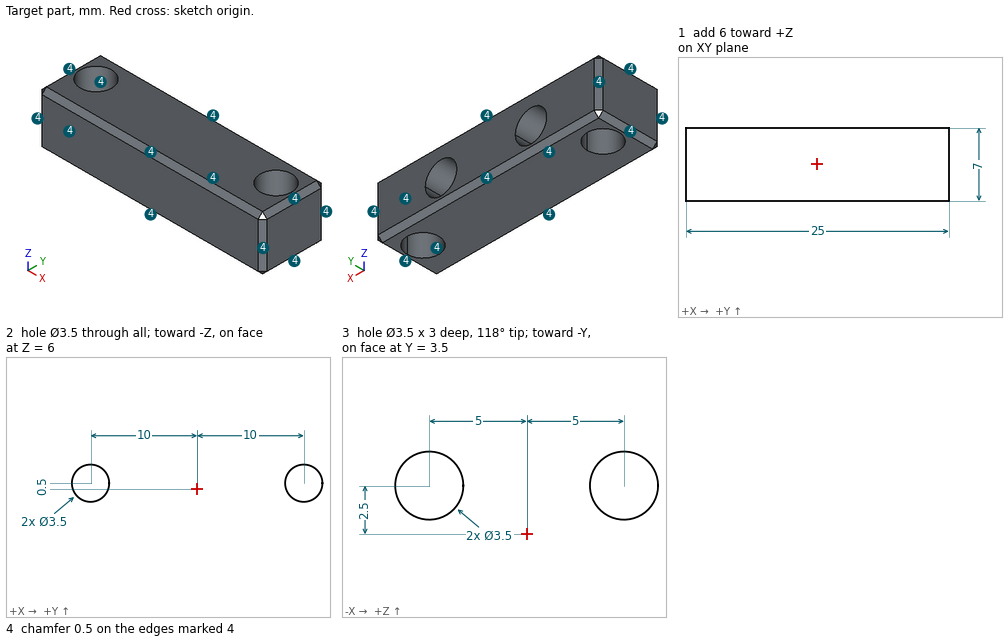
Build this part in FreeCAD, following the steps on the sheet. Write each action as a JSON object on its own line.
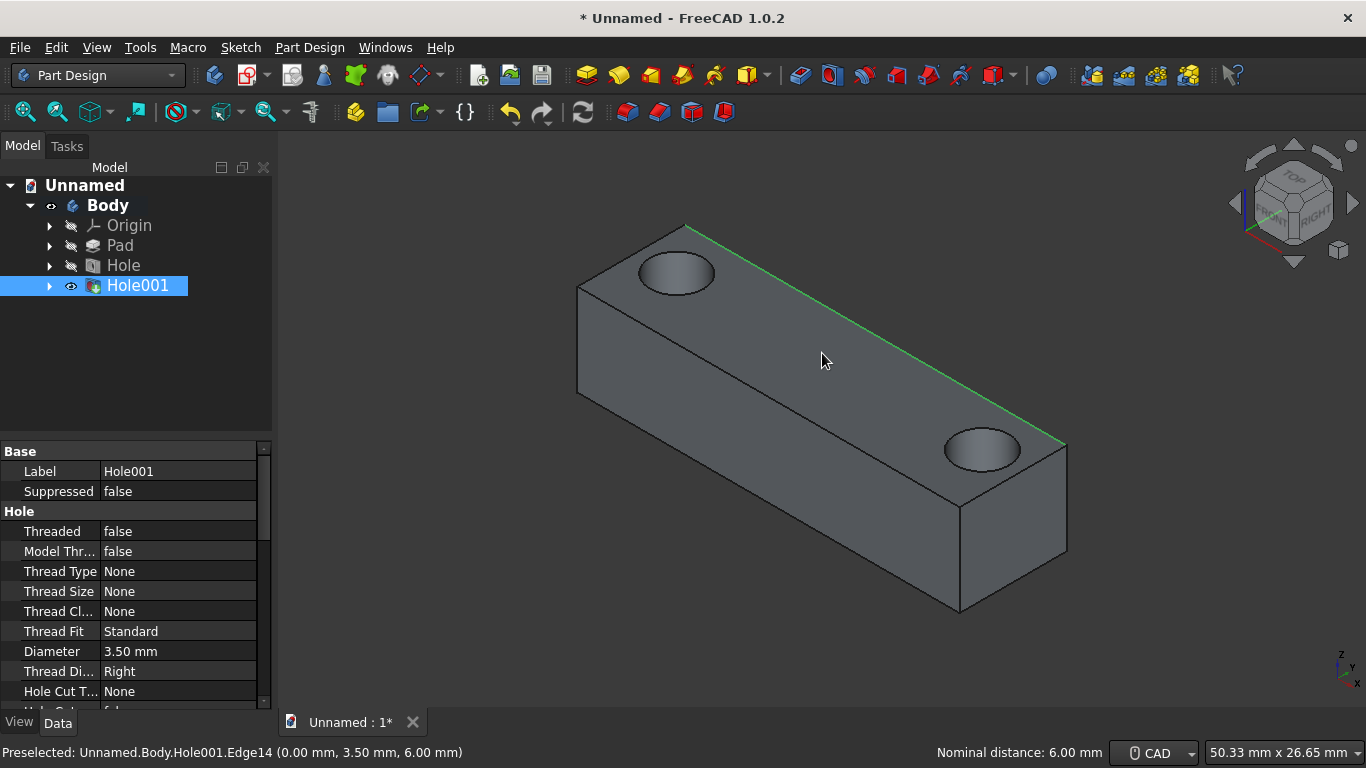
{"action": "left_click", "coordinate": [878, 512], "text": "ctrl"}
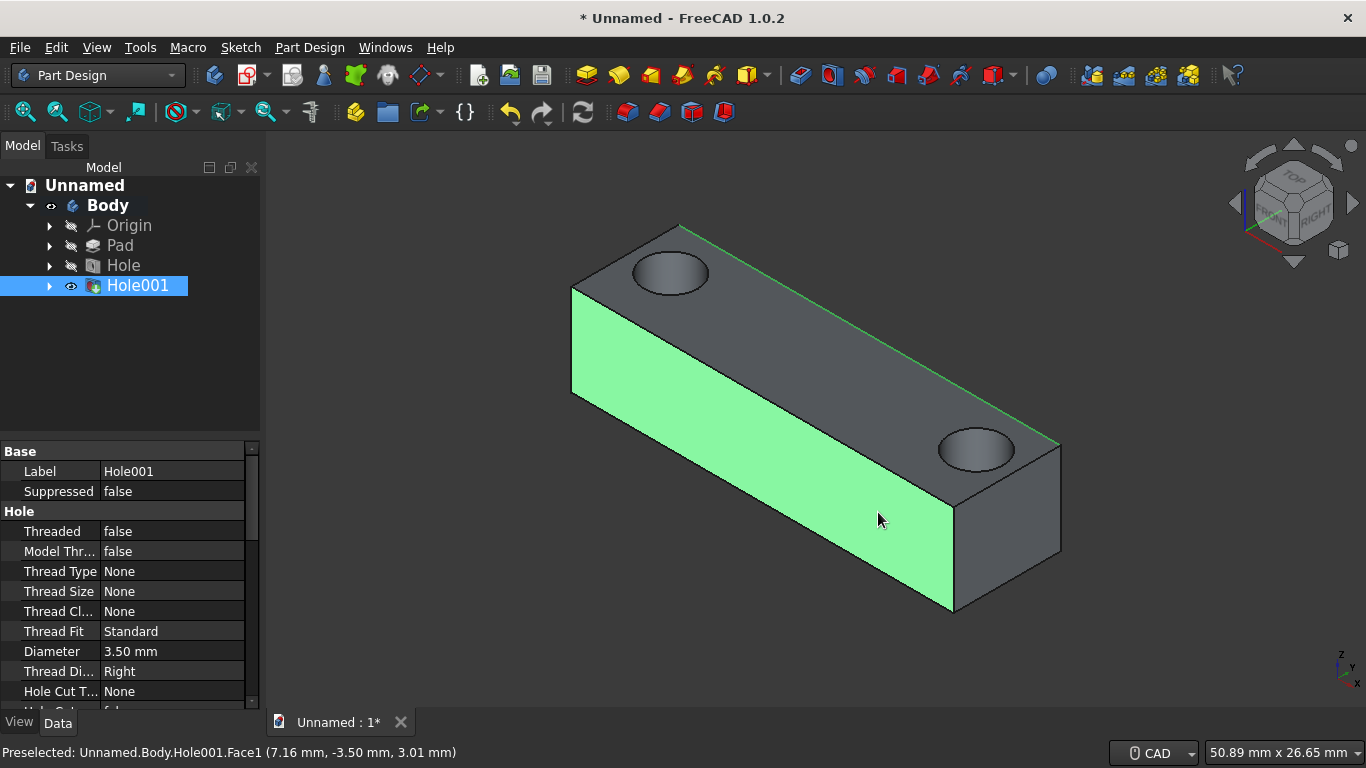
{"action": "left_click", "coordinate": [1007, 528], "text": "ctrl"}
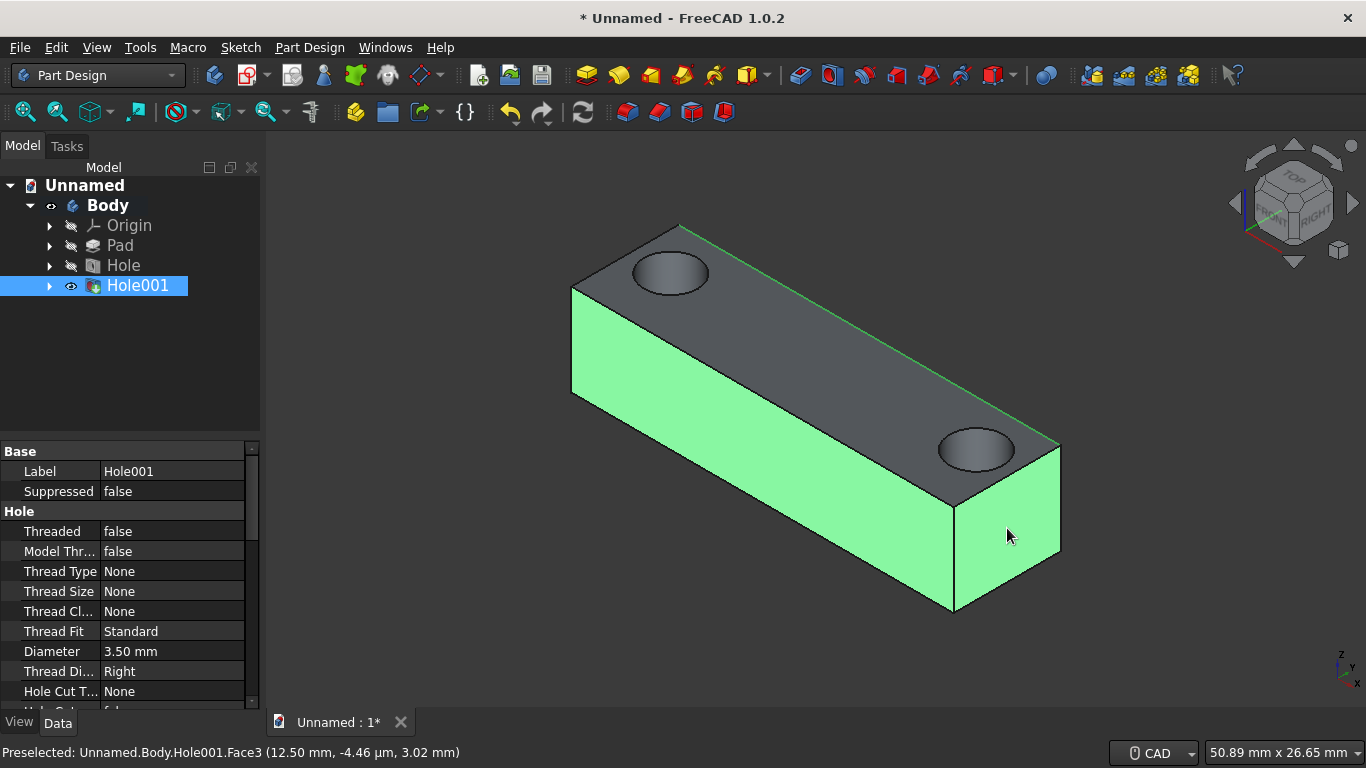
{"action": "key", "text": "2"}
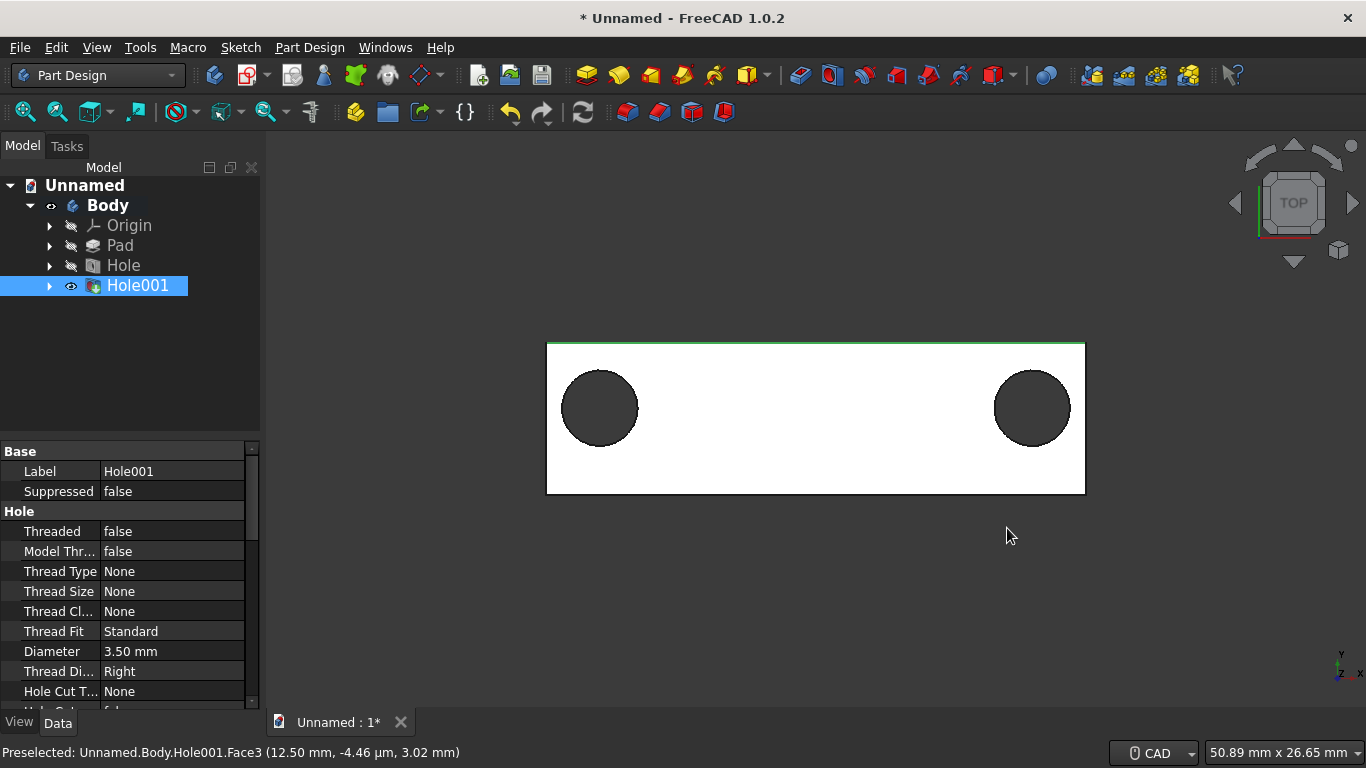
{"action": "key", "text": "1"}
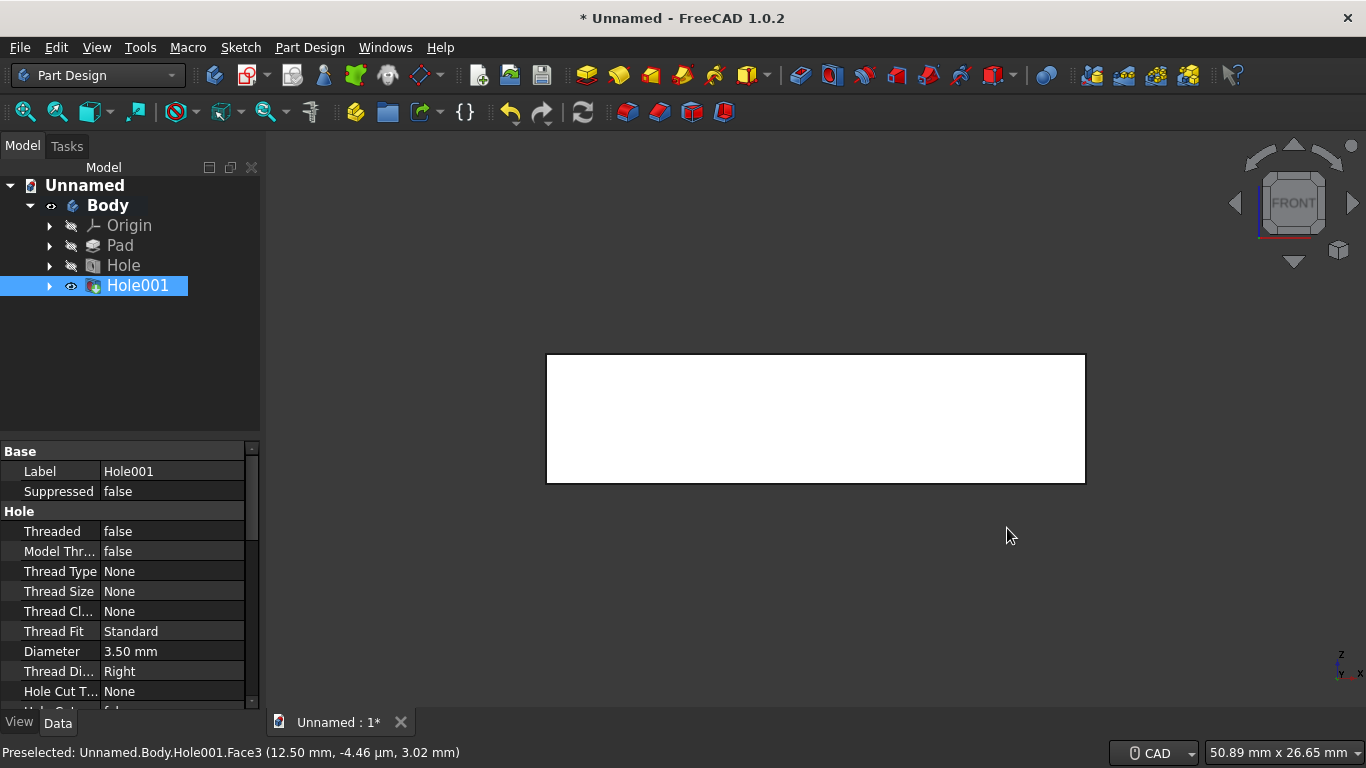
{"action": "key", "text": "3"}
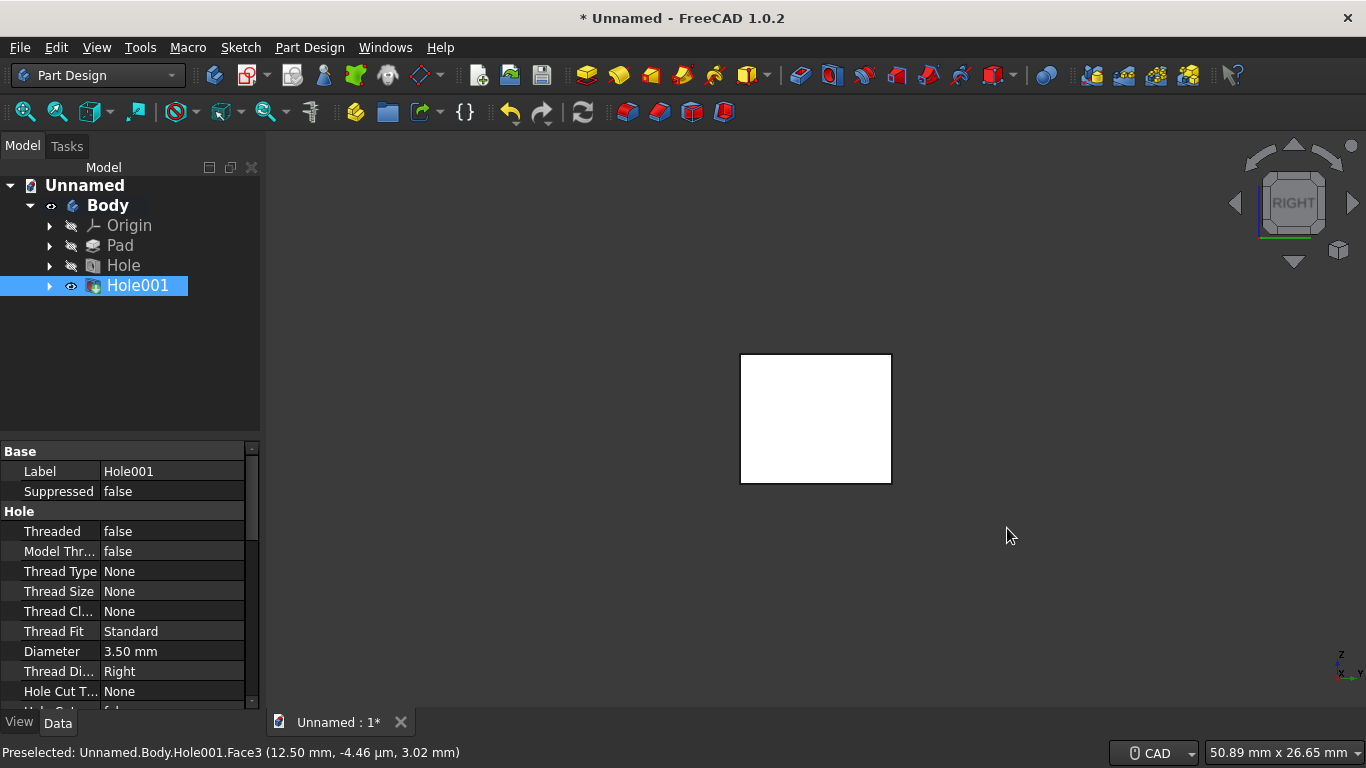
{"action": "left_click", "coordinate": [26, 112]}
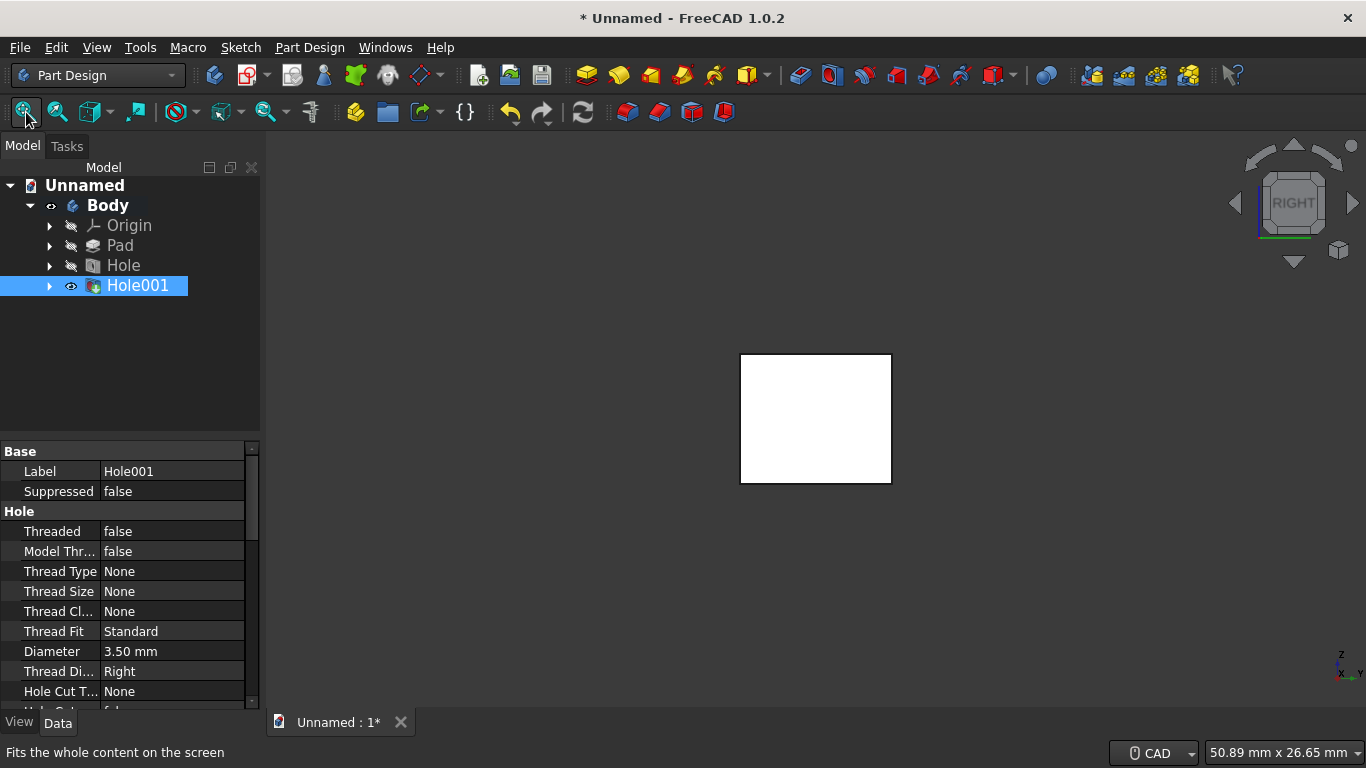
{"action": "key", "text": "5"}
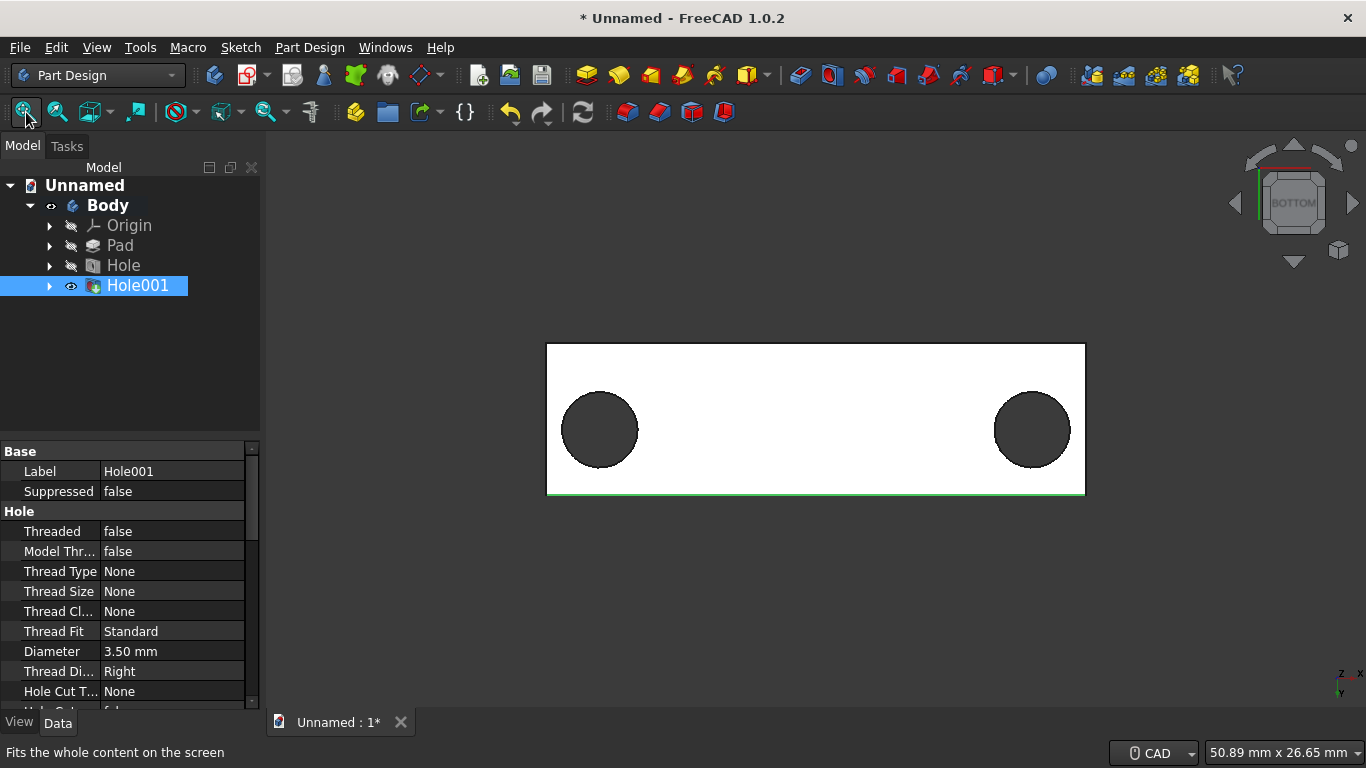
{"action": "key", "text": "4"}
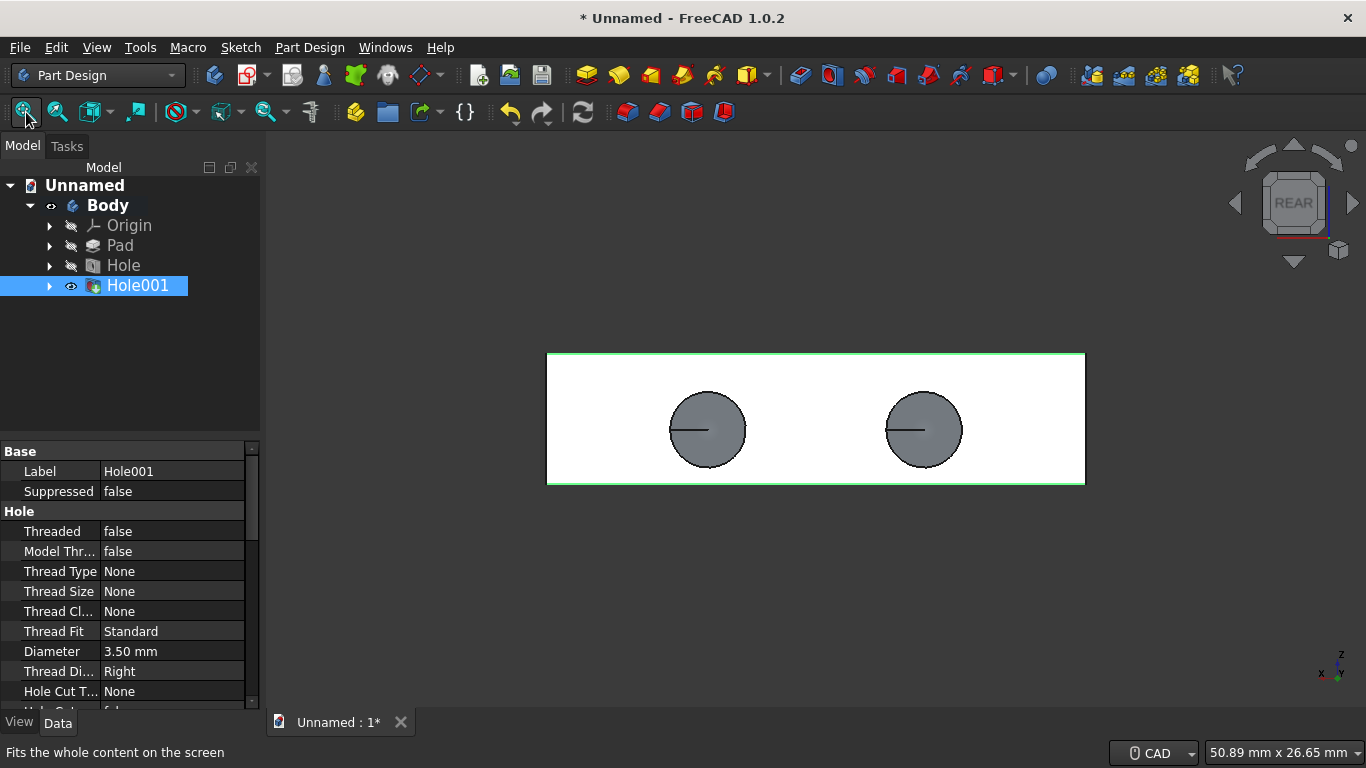
{"action": "key", "text": "6"}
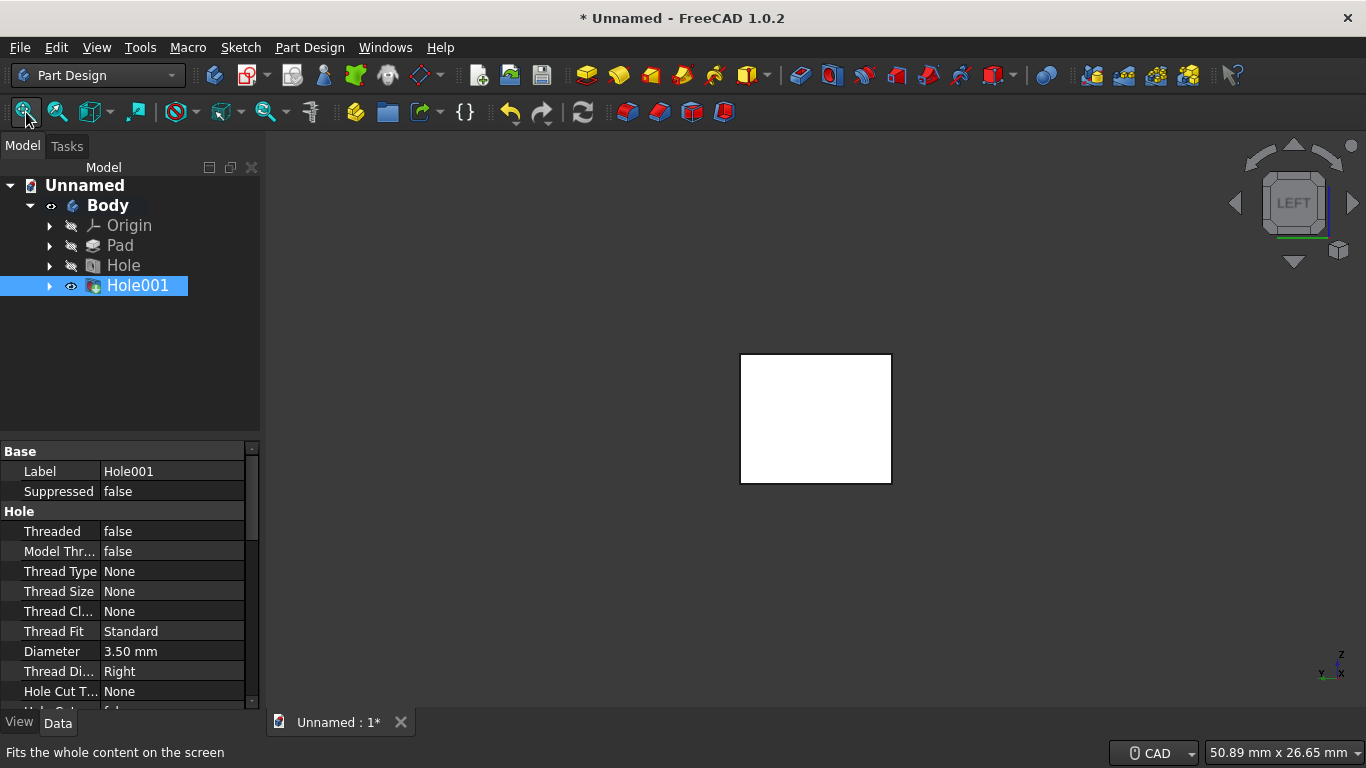
{"action": "left_click", "coordinate": [26, 112]}